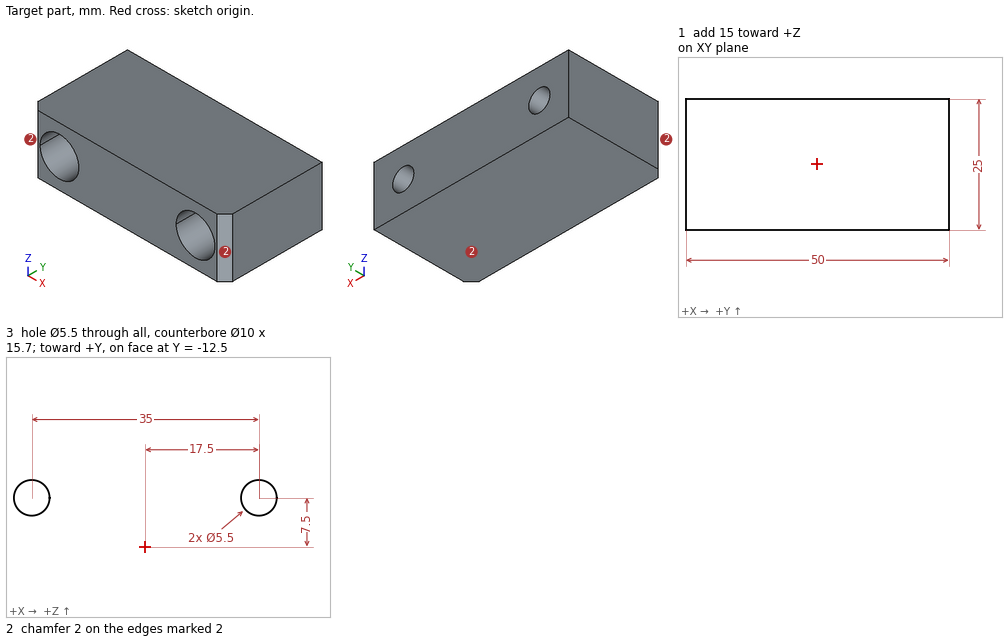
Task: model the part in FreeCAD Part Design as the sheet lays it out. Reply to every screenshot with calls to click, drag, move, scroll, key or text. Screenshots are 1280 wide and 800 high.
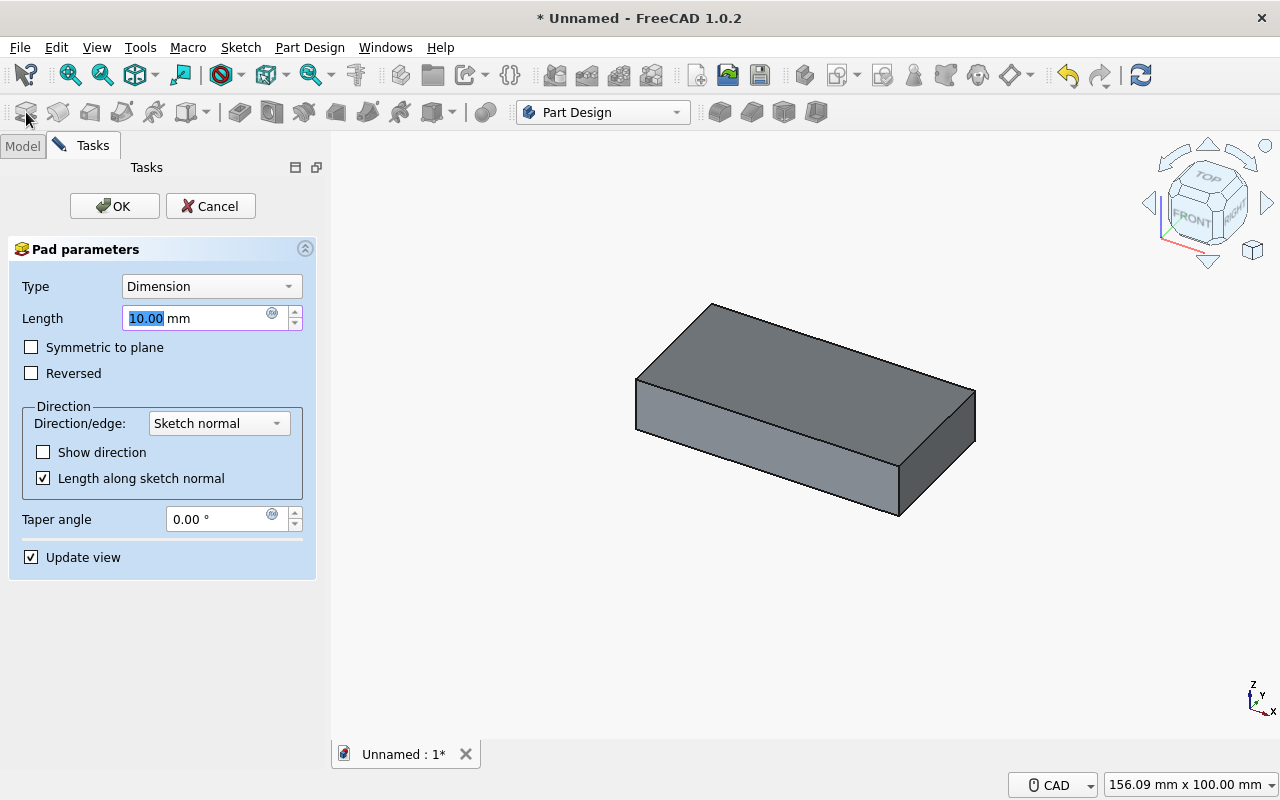
text(15)
key(Tab)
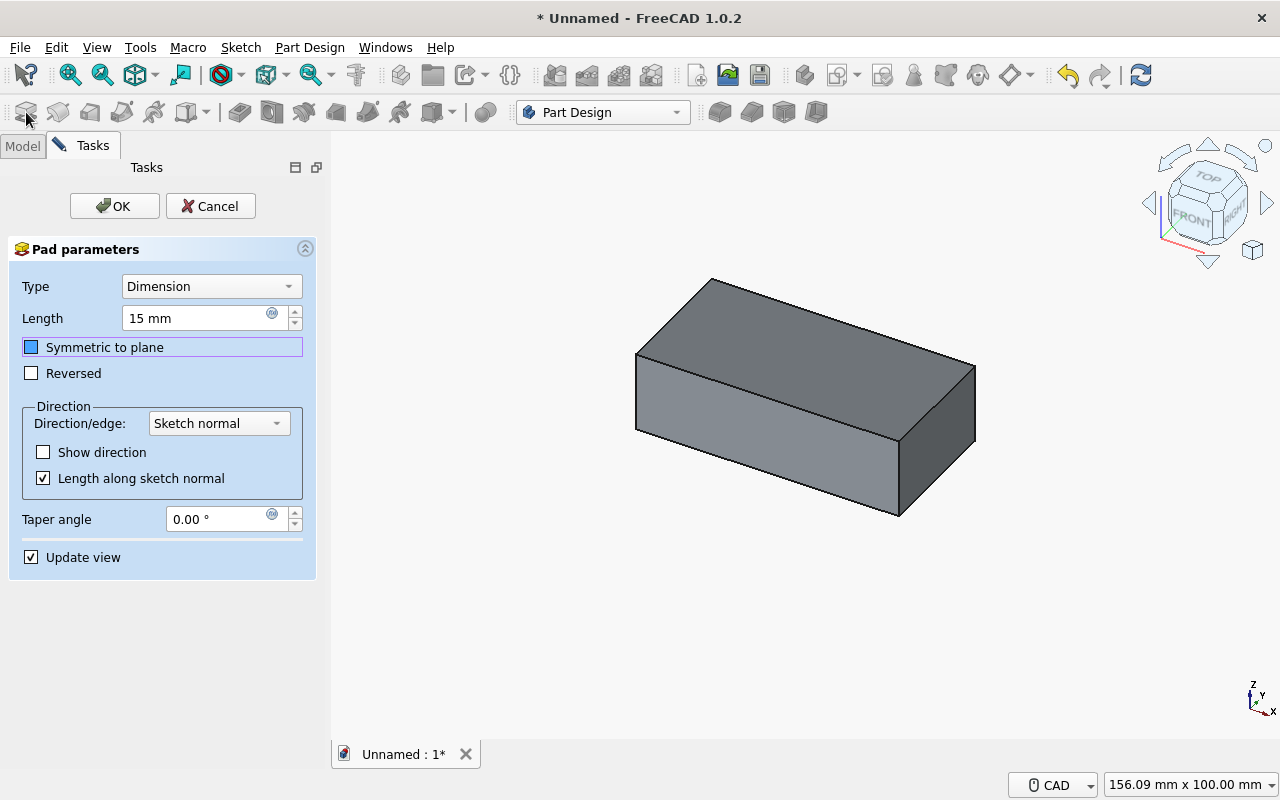
click(115, 206)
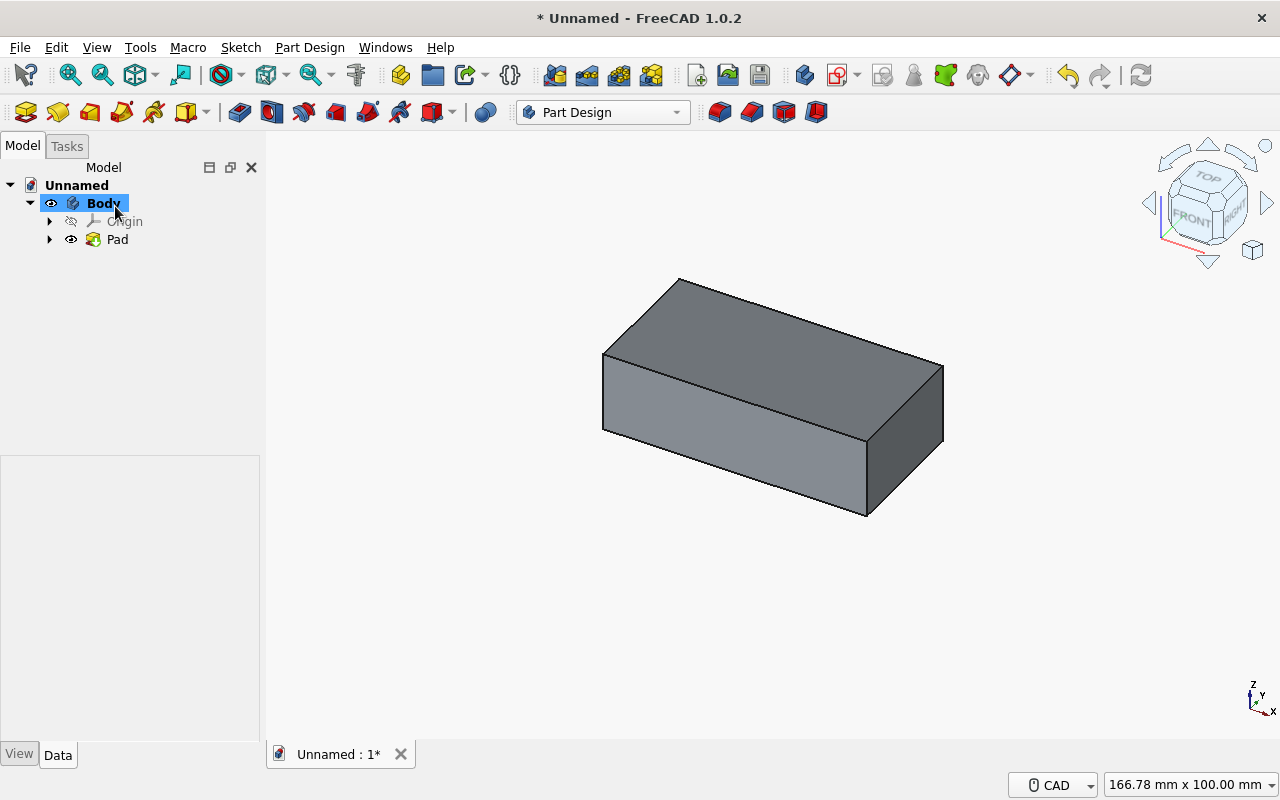
key(v)
key(f)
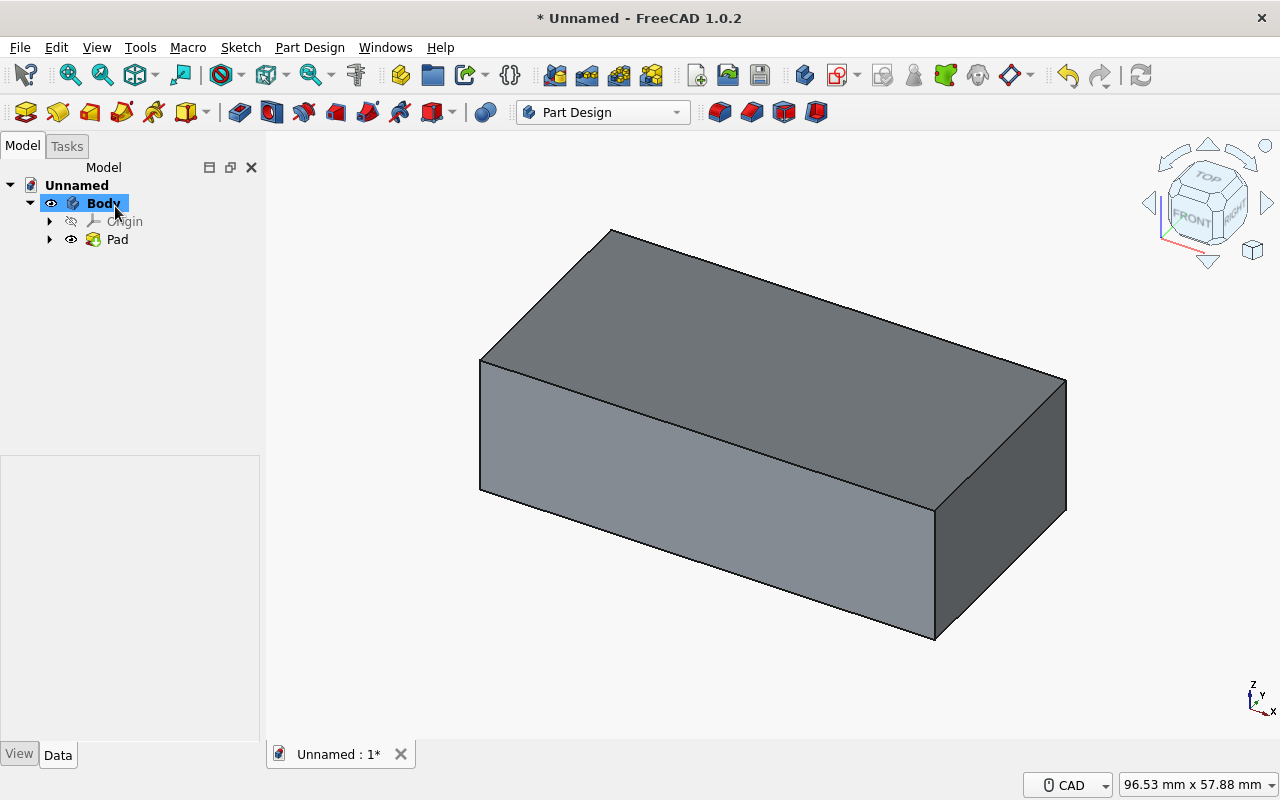
click(935, 575)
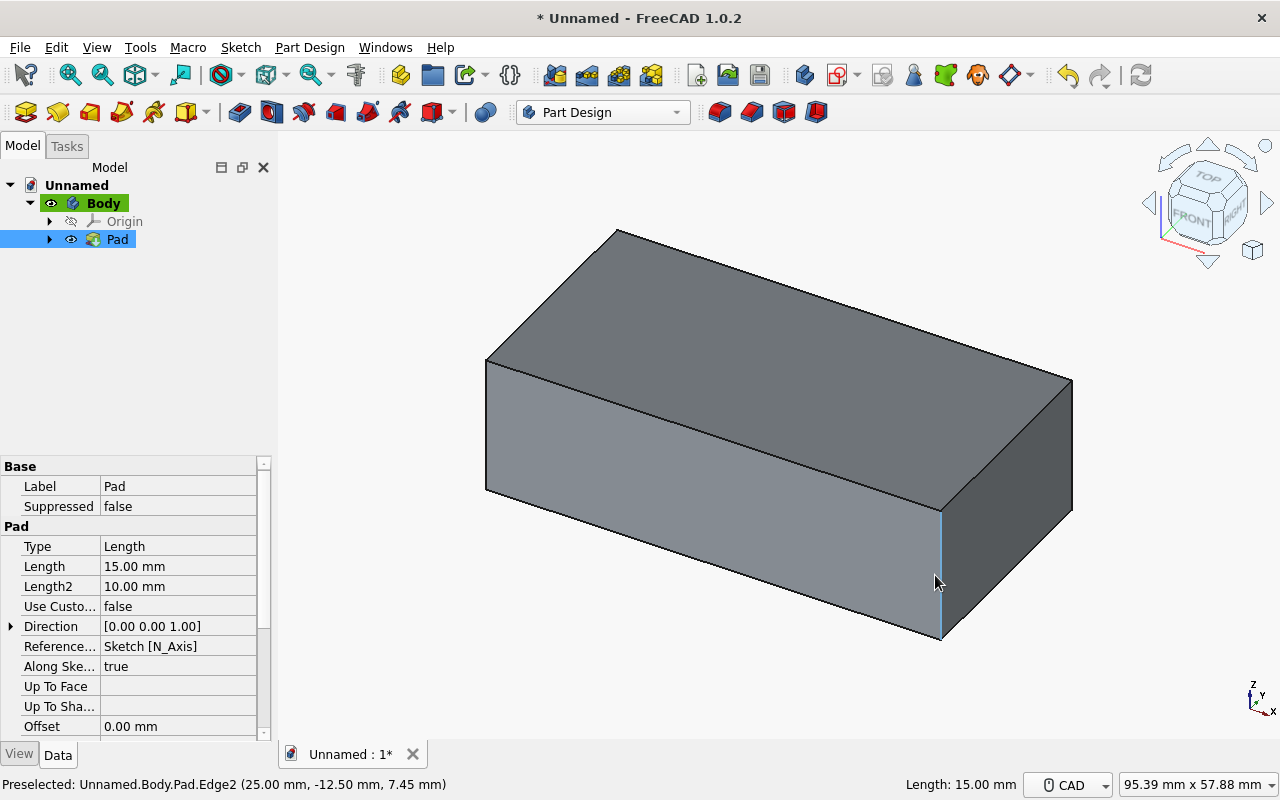
key(0)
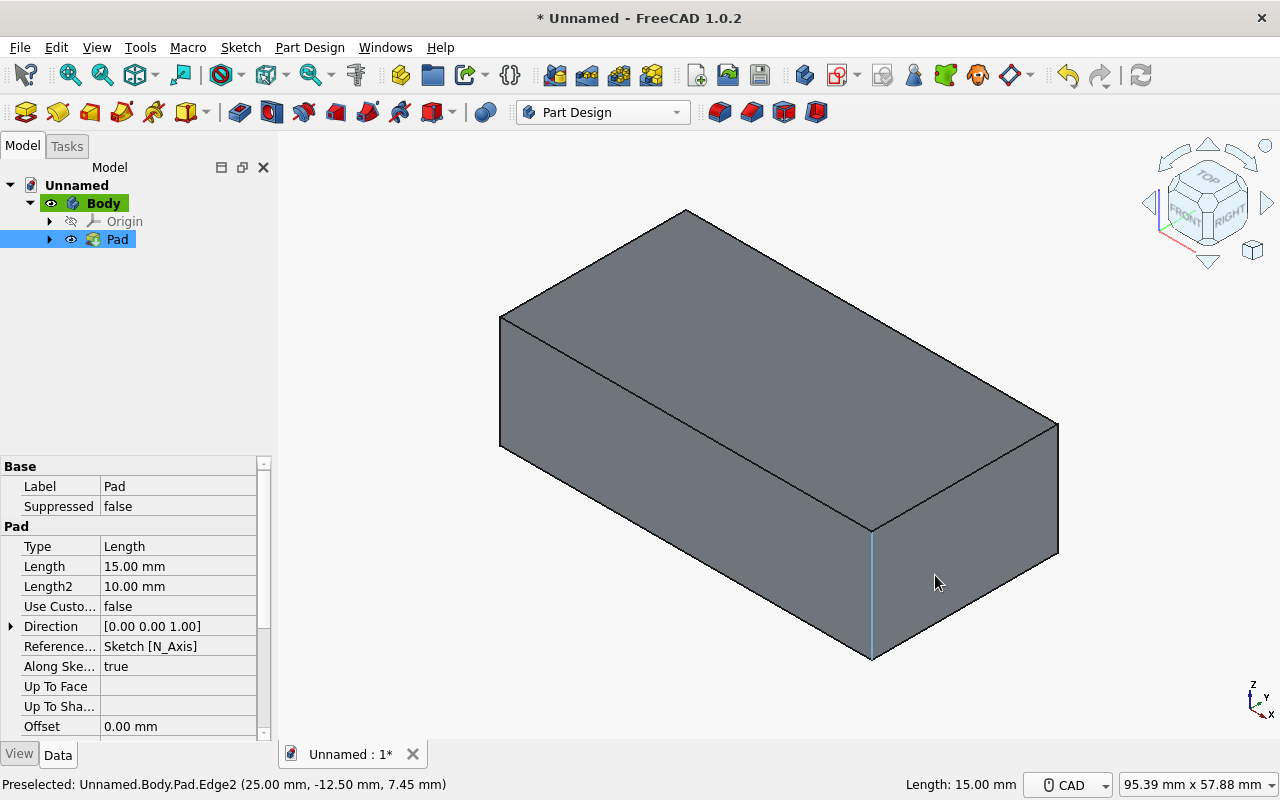
key(2)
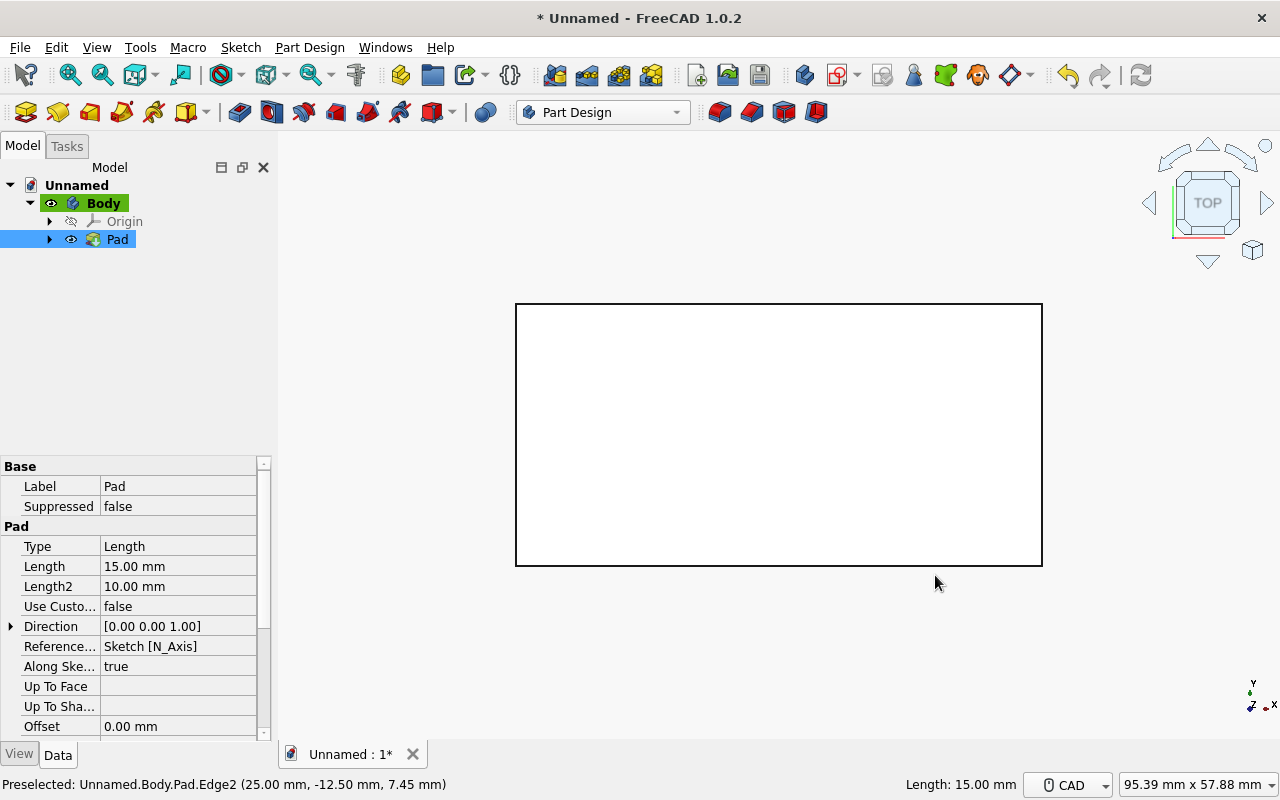
key(1)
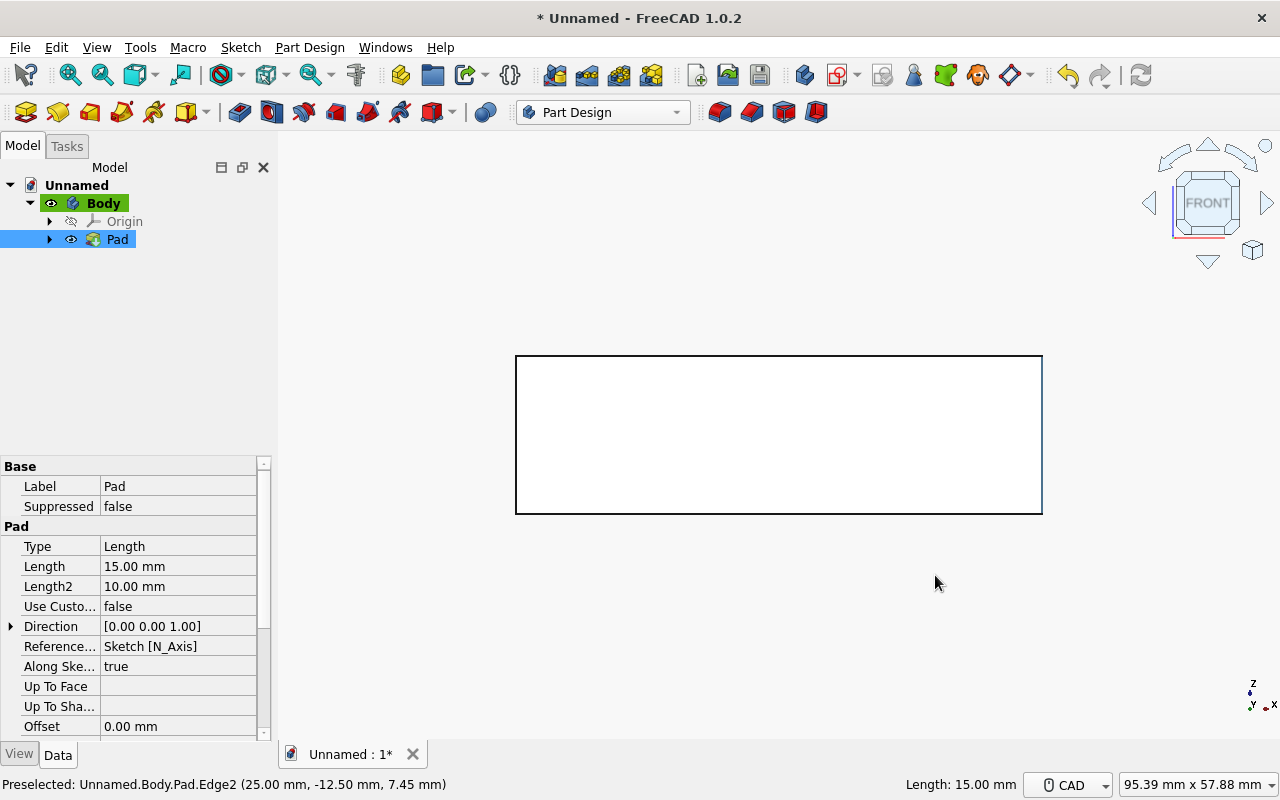
click(516, 434, ctrl)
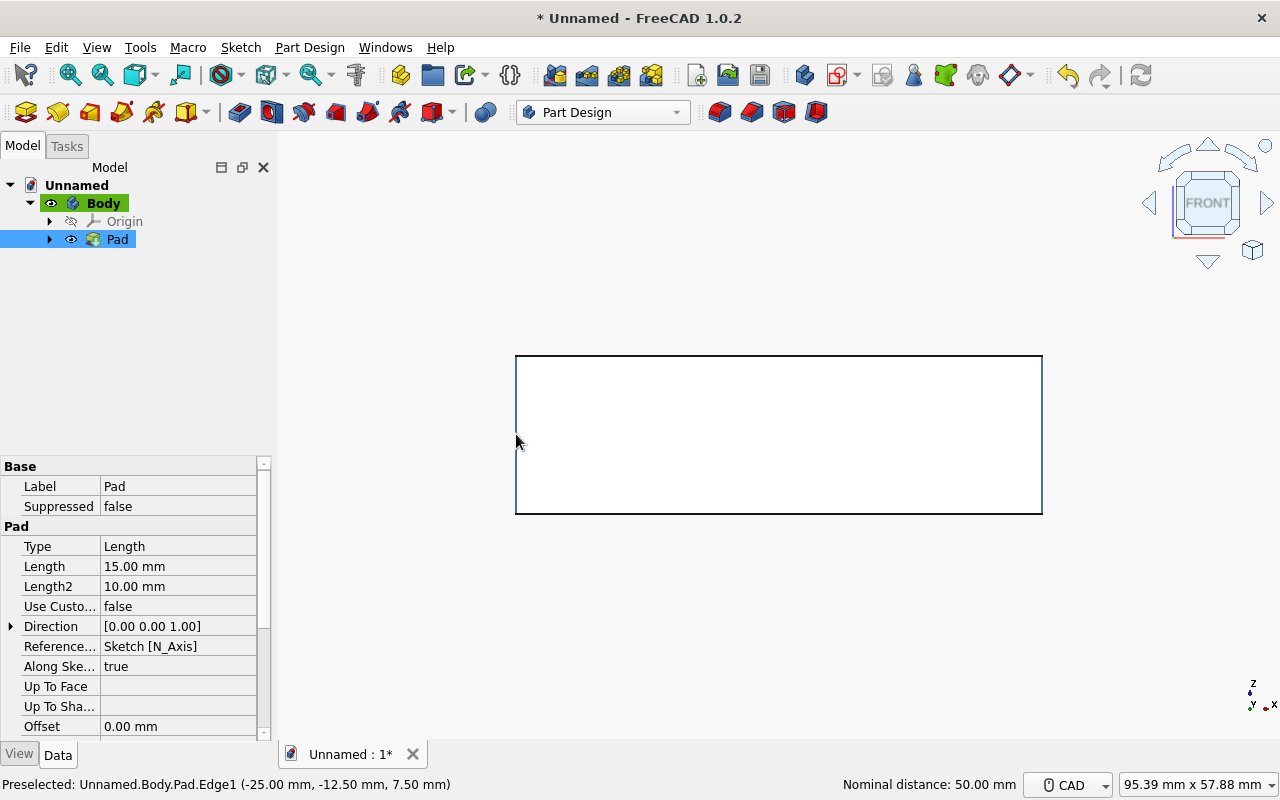
click(752, 112)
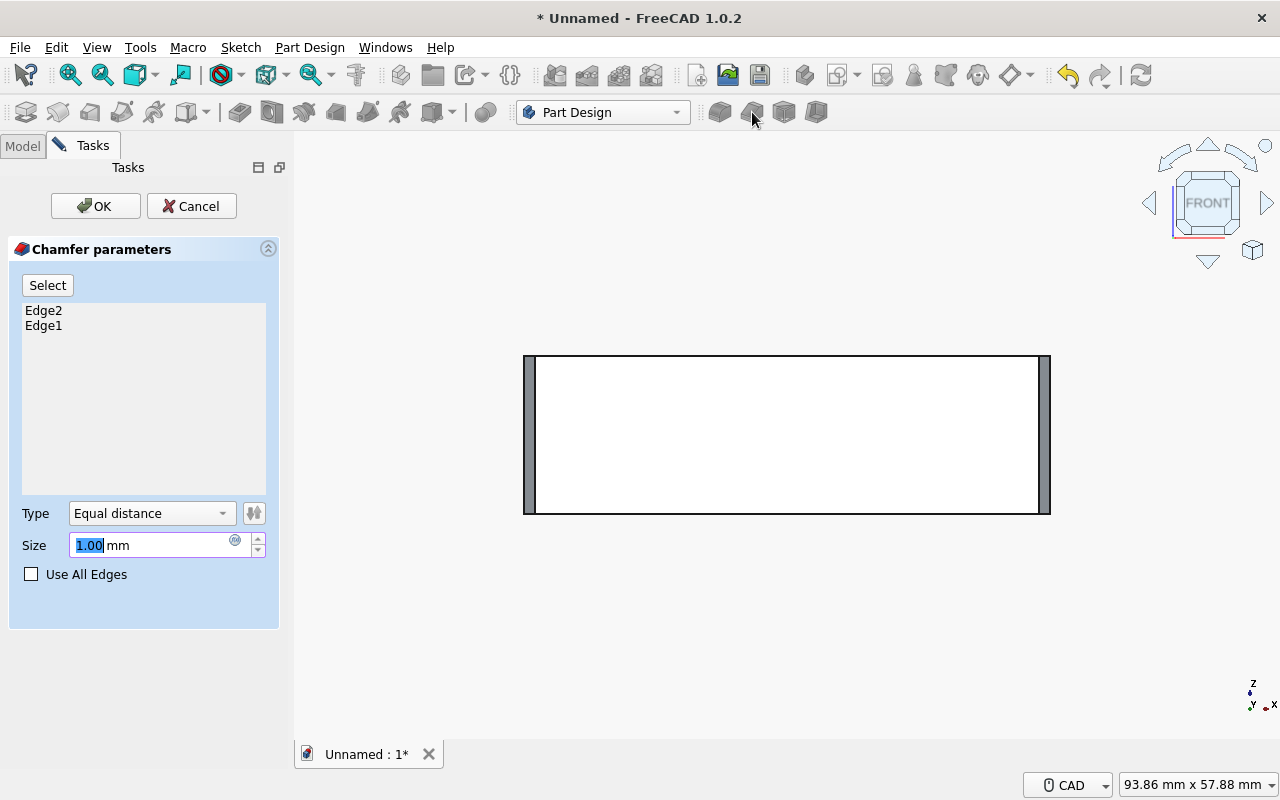
text(2)
key(Tab)